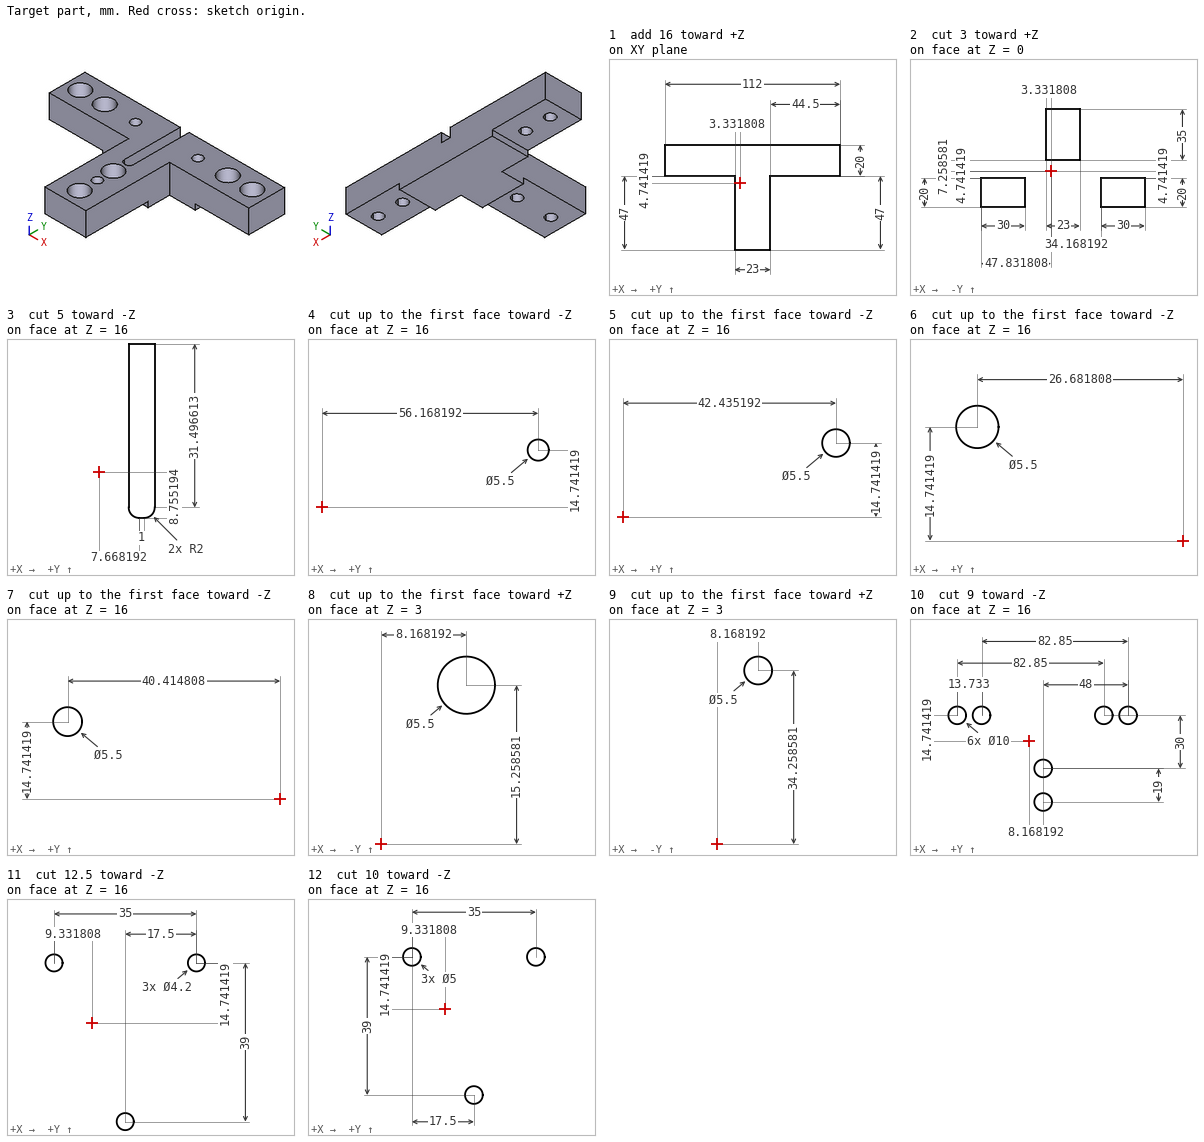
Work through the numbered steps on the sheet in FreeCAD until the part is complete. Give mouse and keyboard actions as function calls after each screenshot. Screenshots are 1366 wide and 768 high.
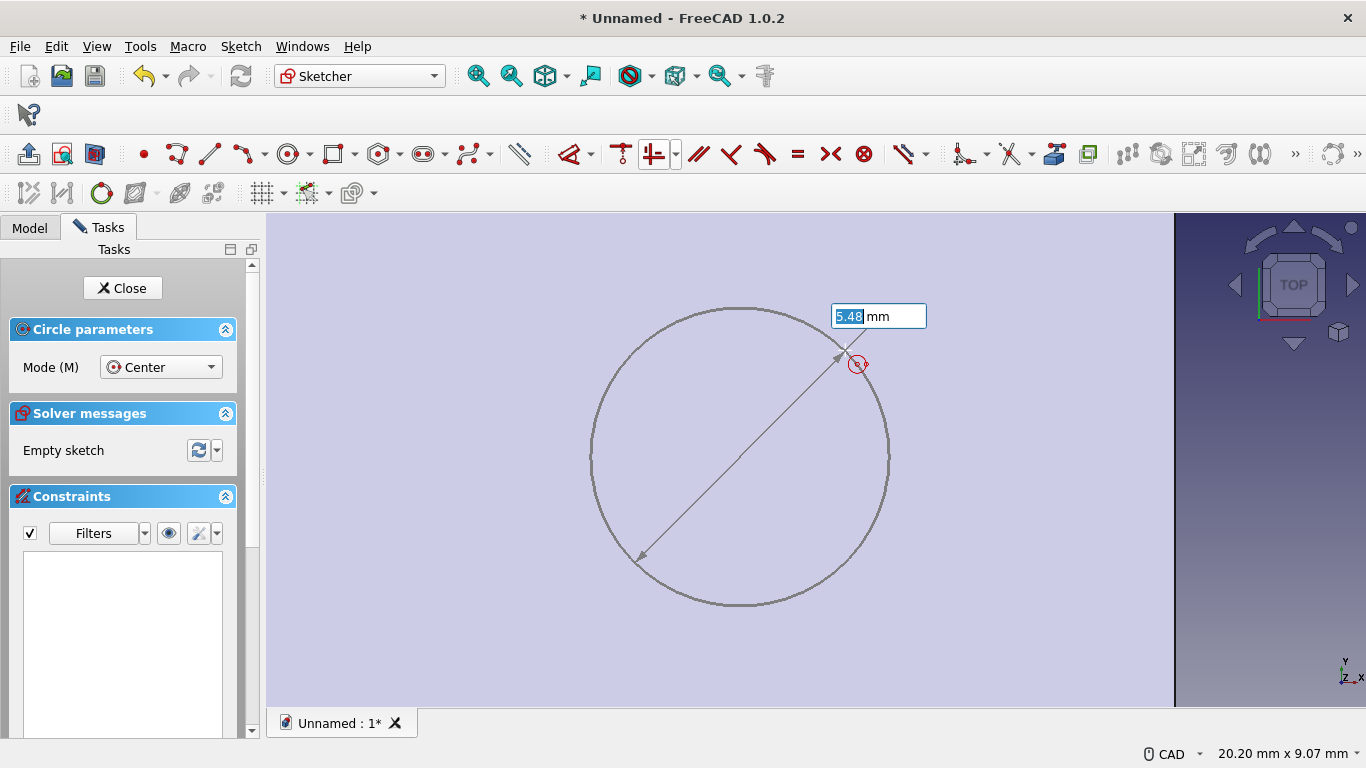
text(5.5)
key(Return)
key(Escape)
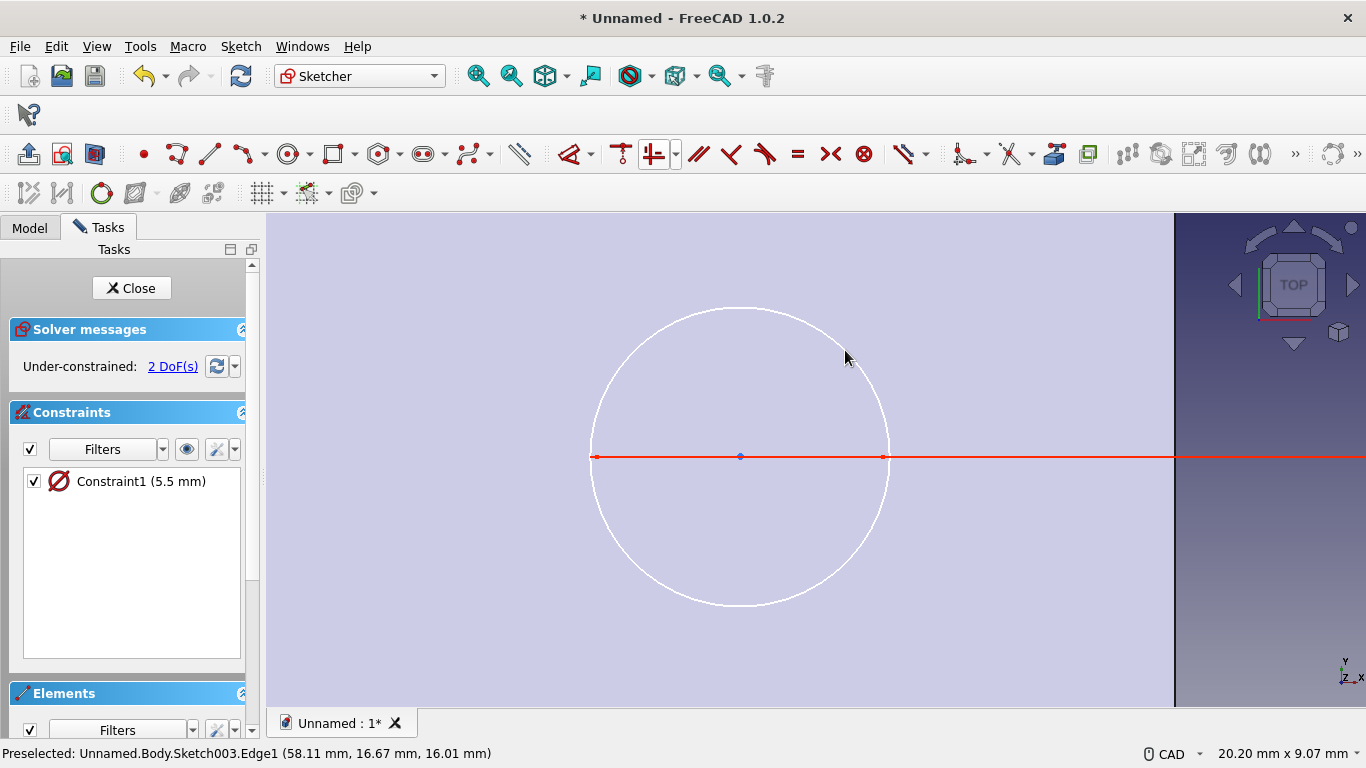
click(568, 154)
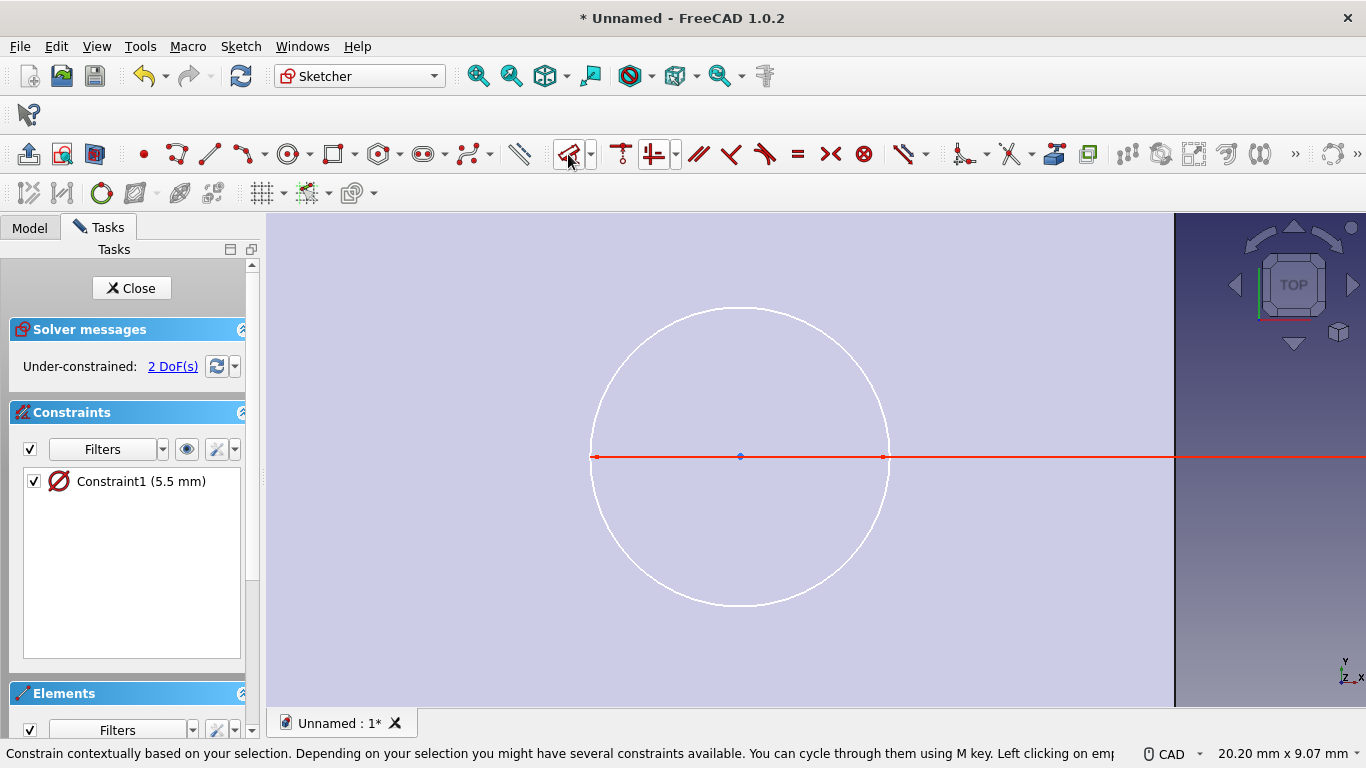
click(740, 457)
click(517, 423)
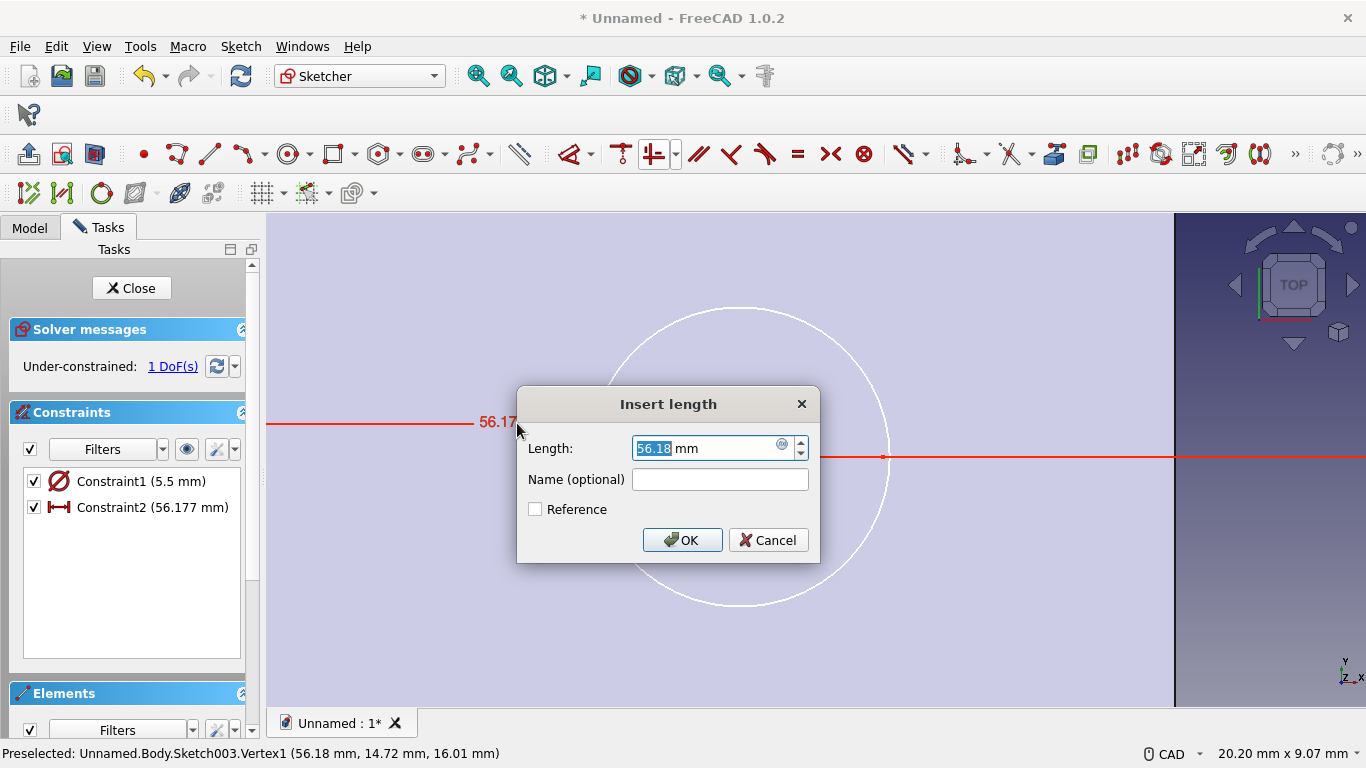
text(56.168192)
key(Return)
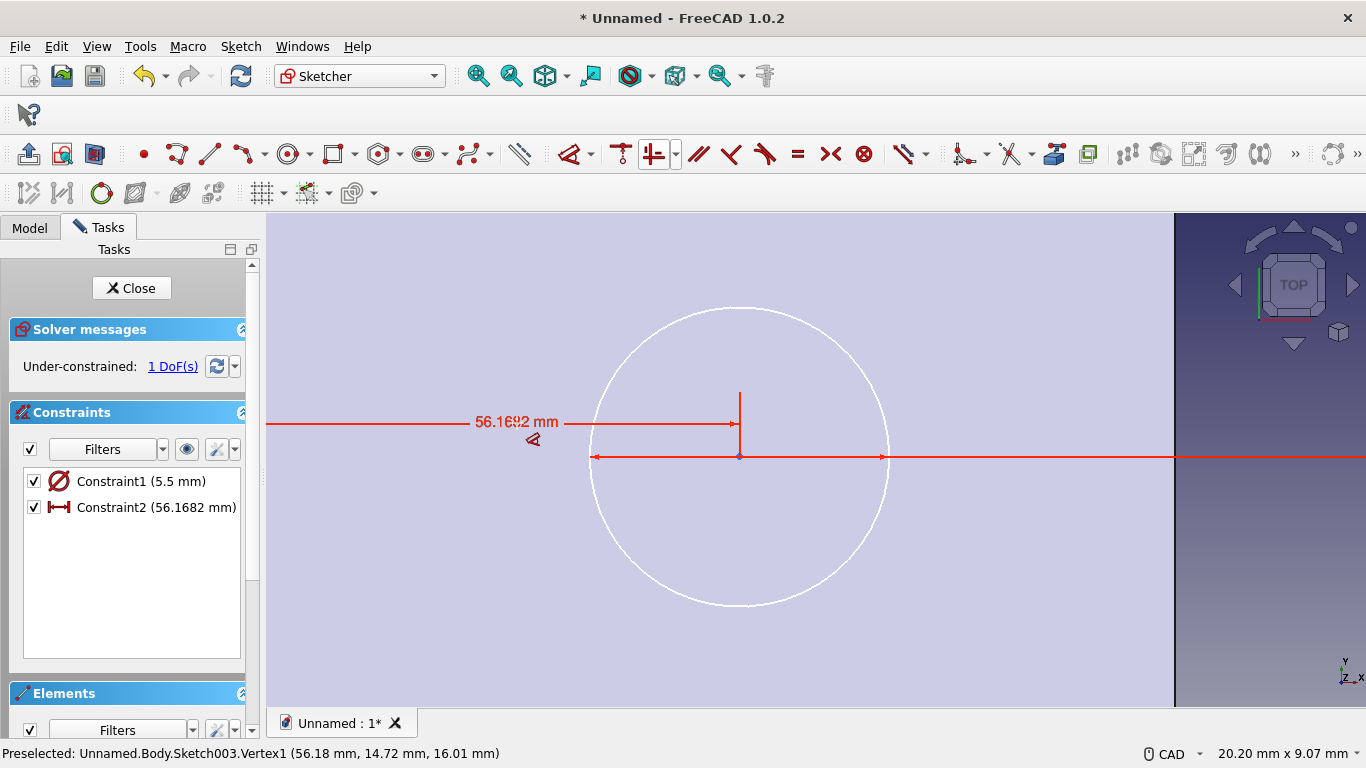
click(740, 457)
click(774, 568)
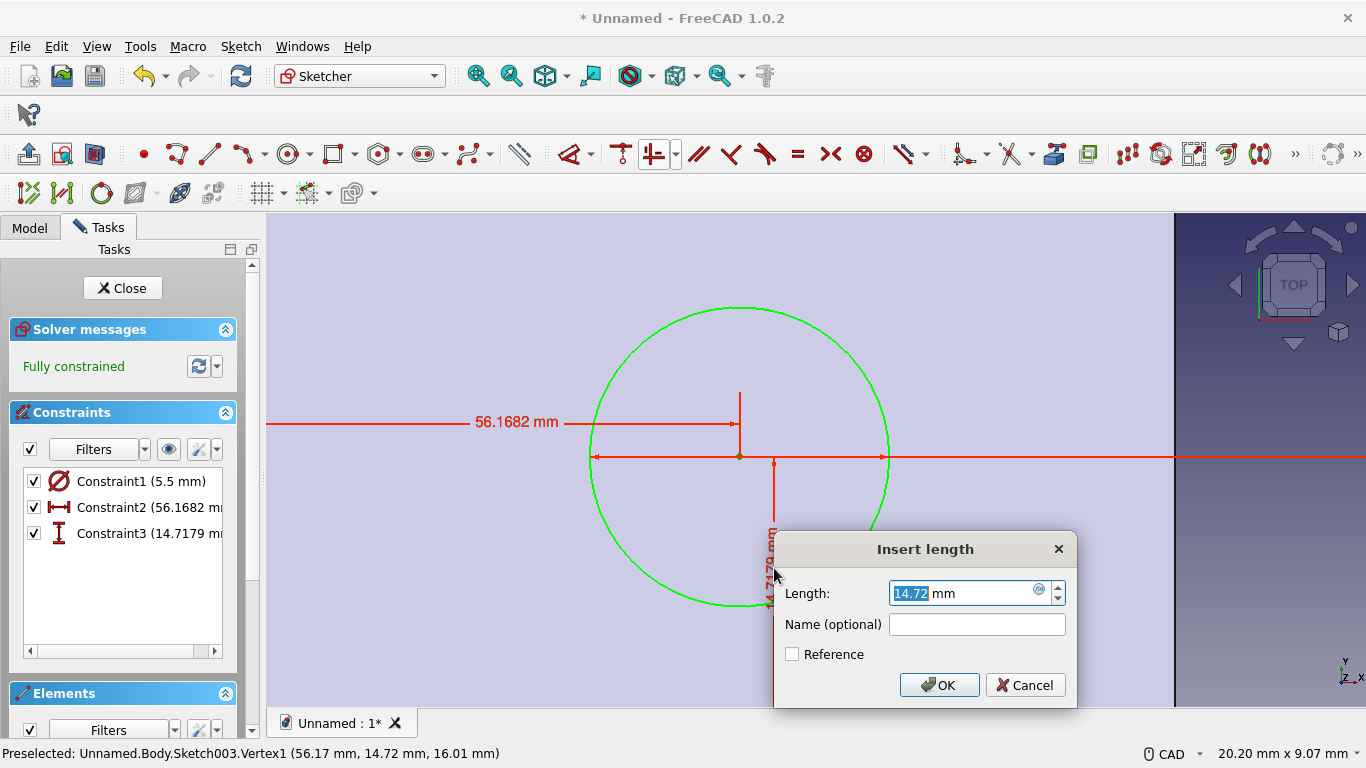
text(14.741419)
key(Return)
key(Escape)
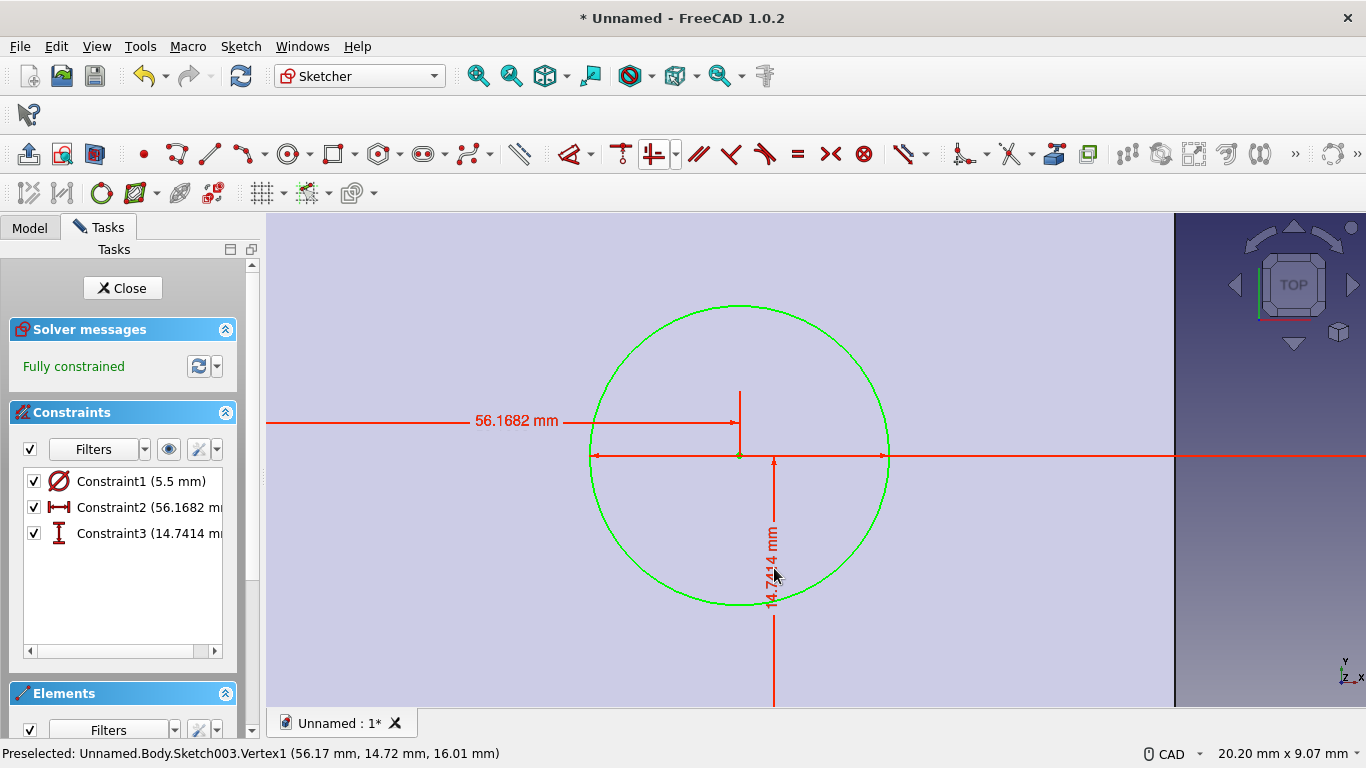
click(123, 288)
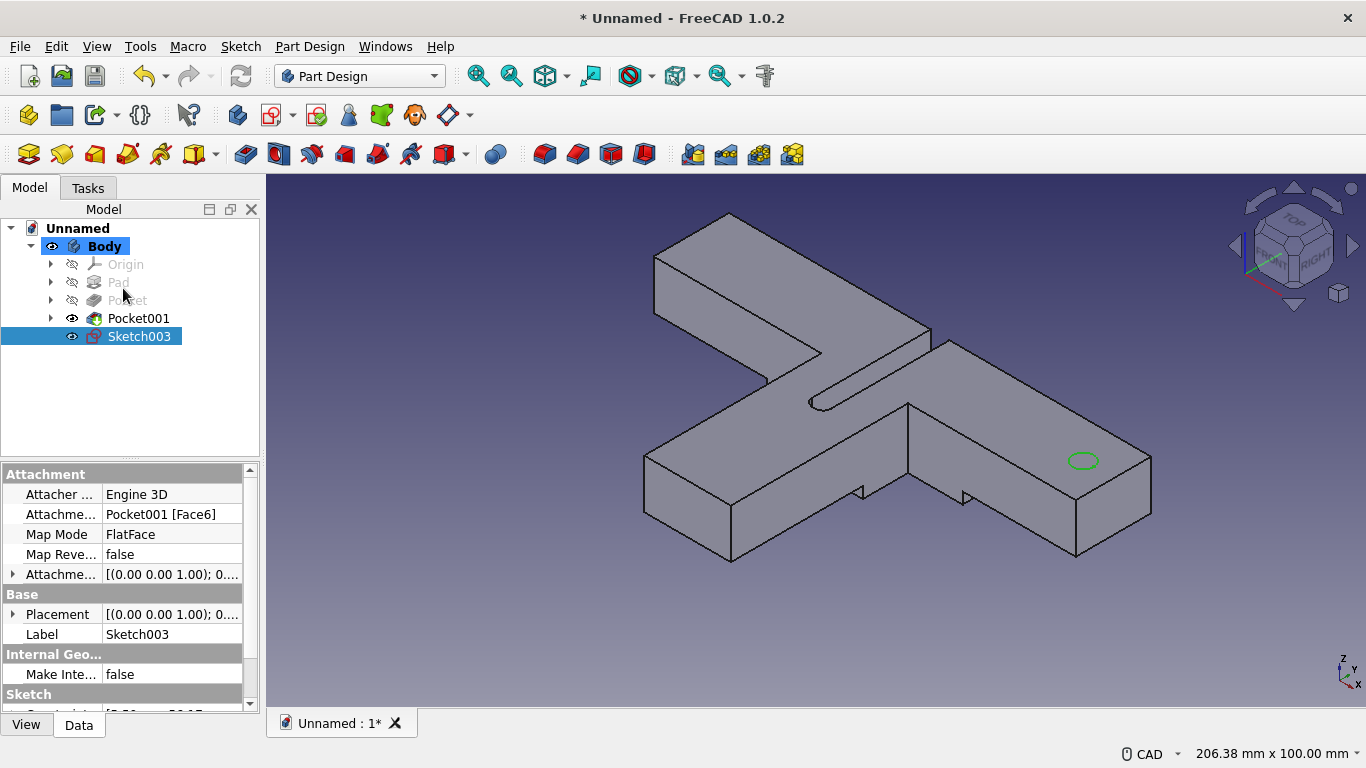
click(246, 154)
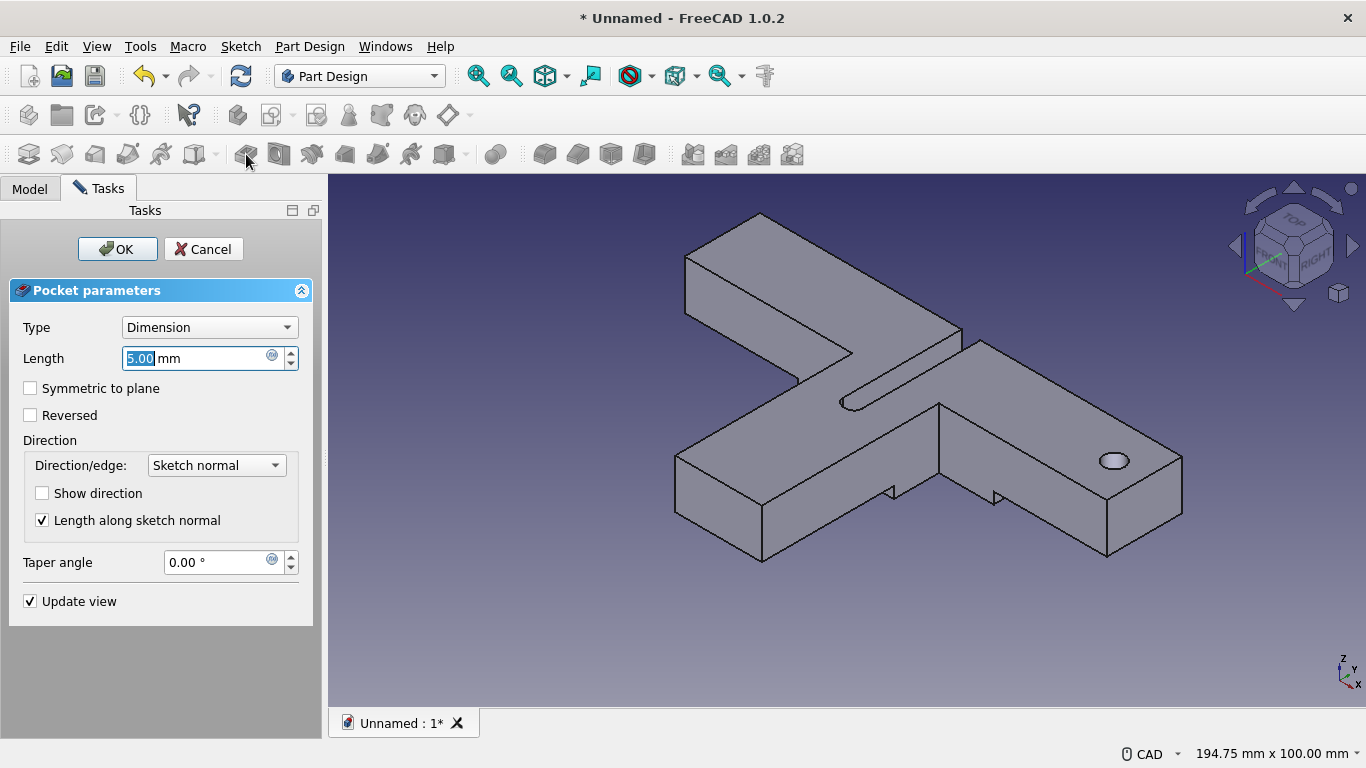
click(210, 328)